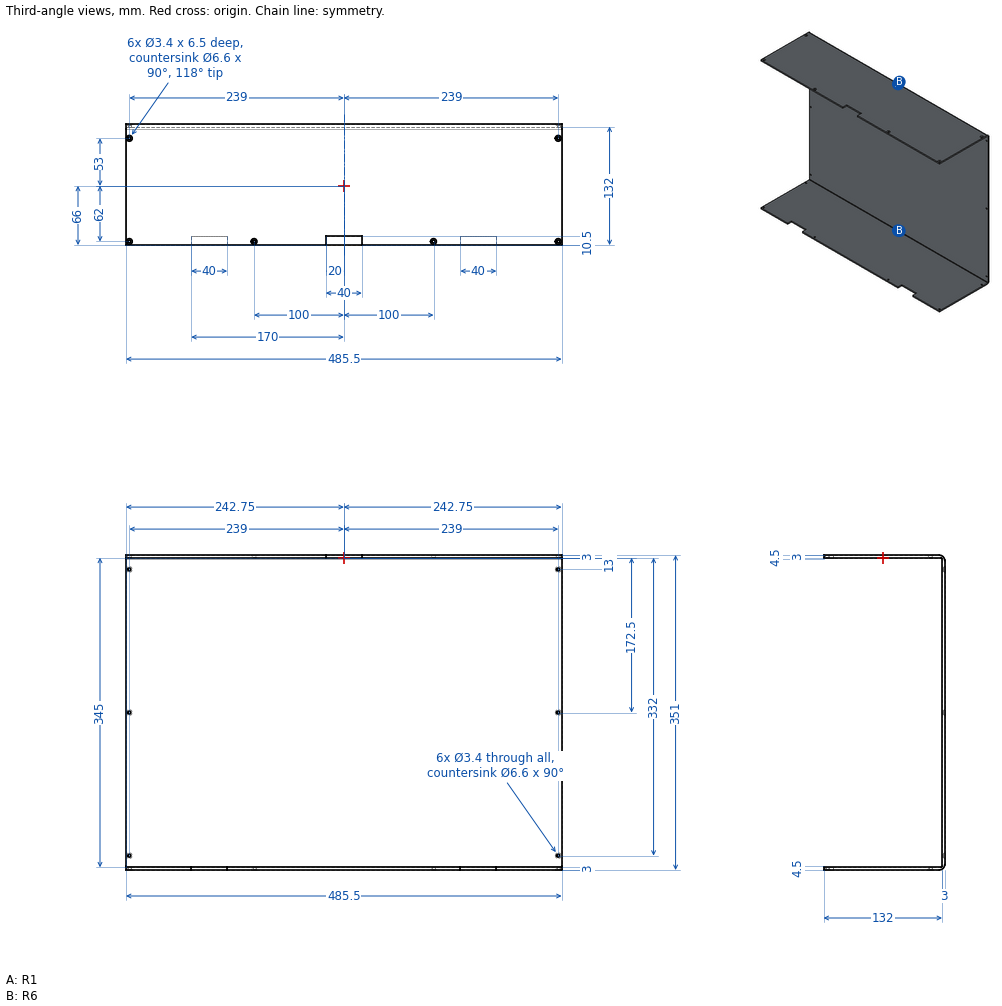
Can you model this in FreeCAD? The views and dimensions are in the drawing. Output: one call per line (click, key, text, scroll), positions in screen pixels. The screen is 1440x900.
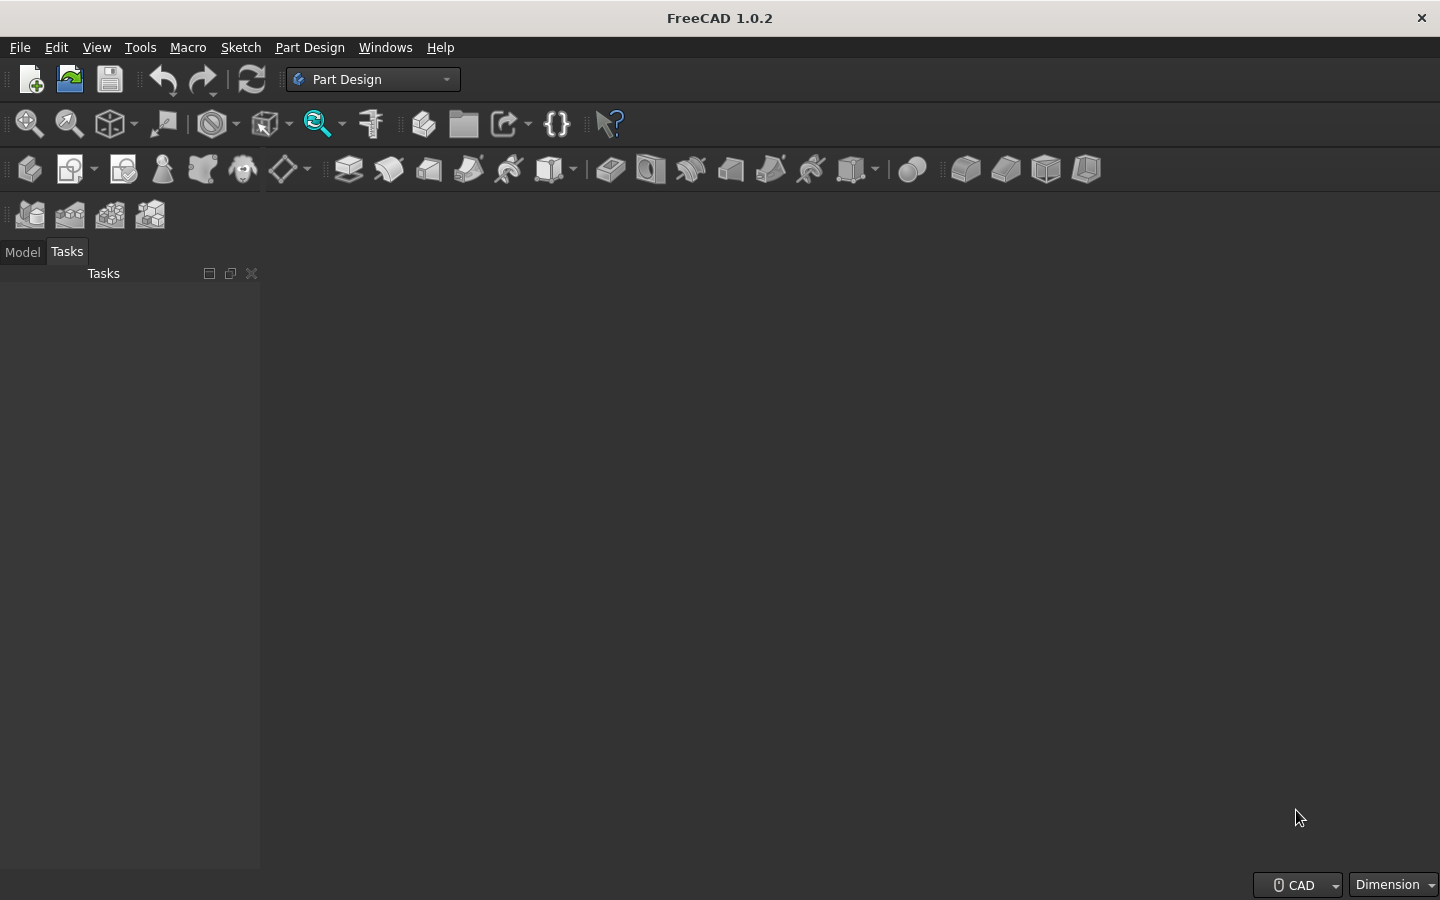
click(1214, 80)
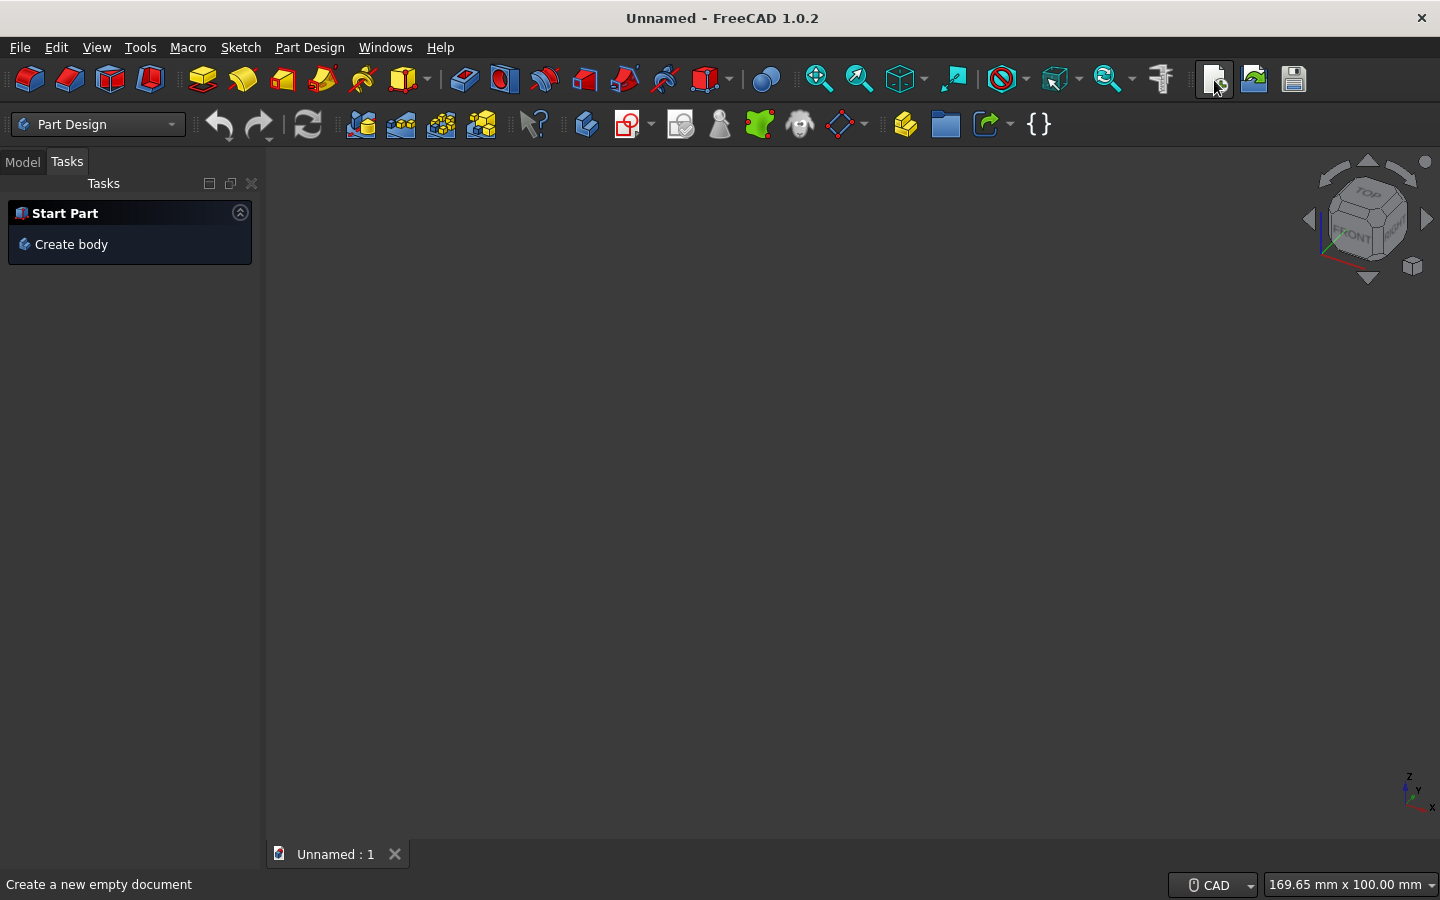
click(628, 124)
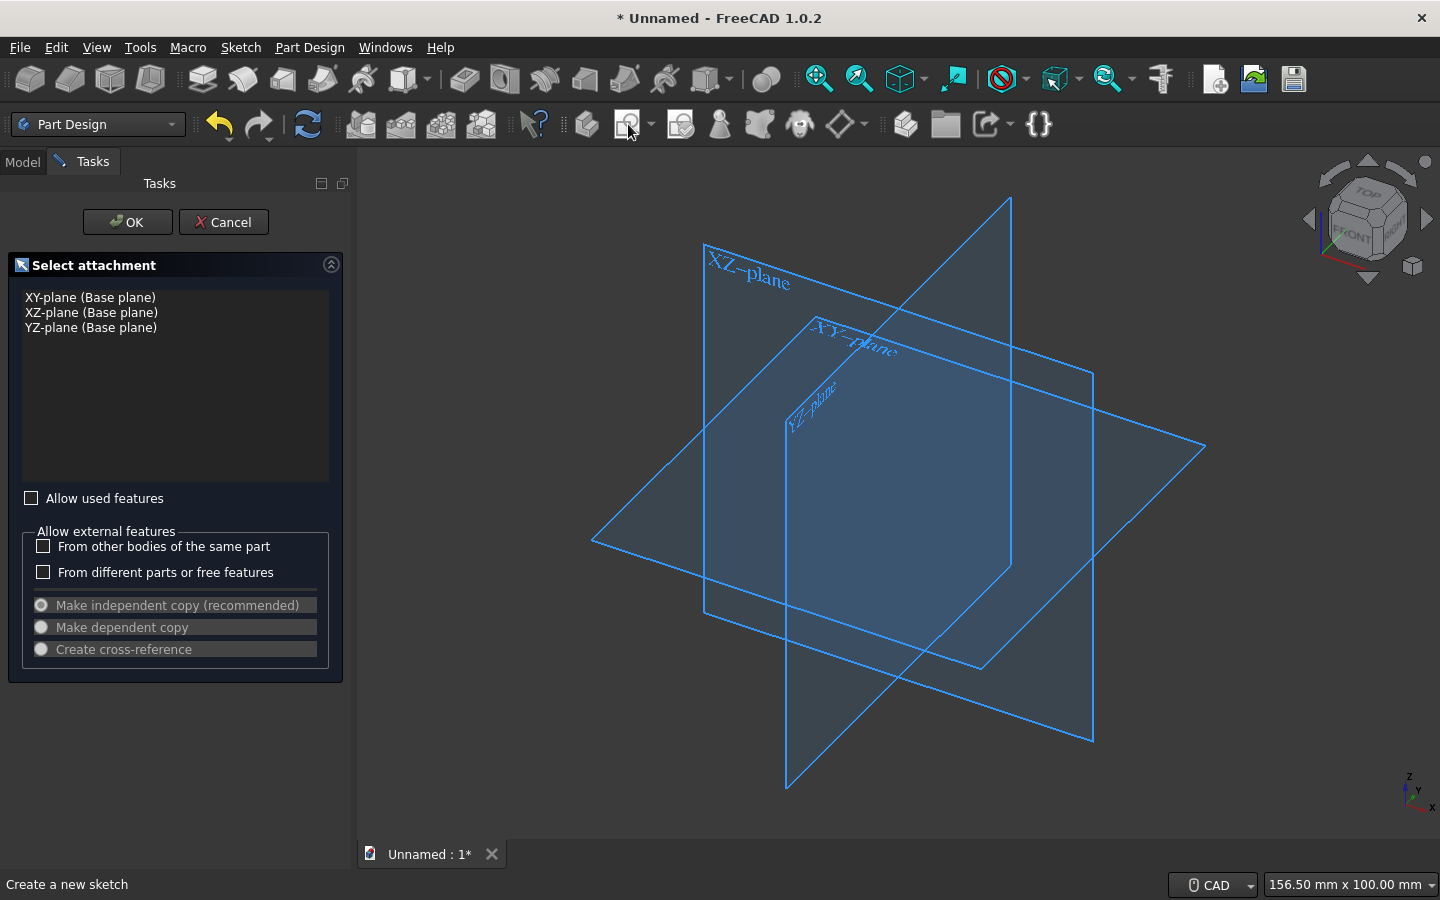
click(82, 298)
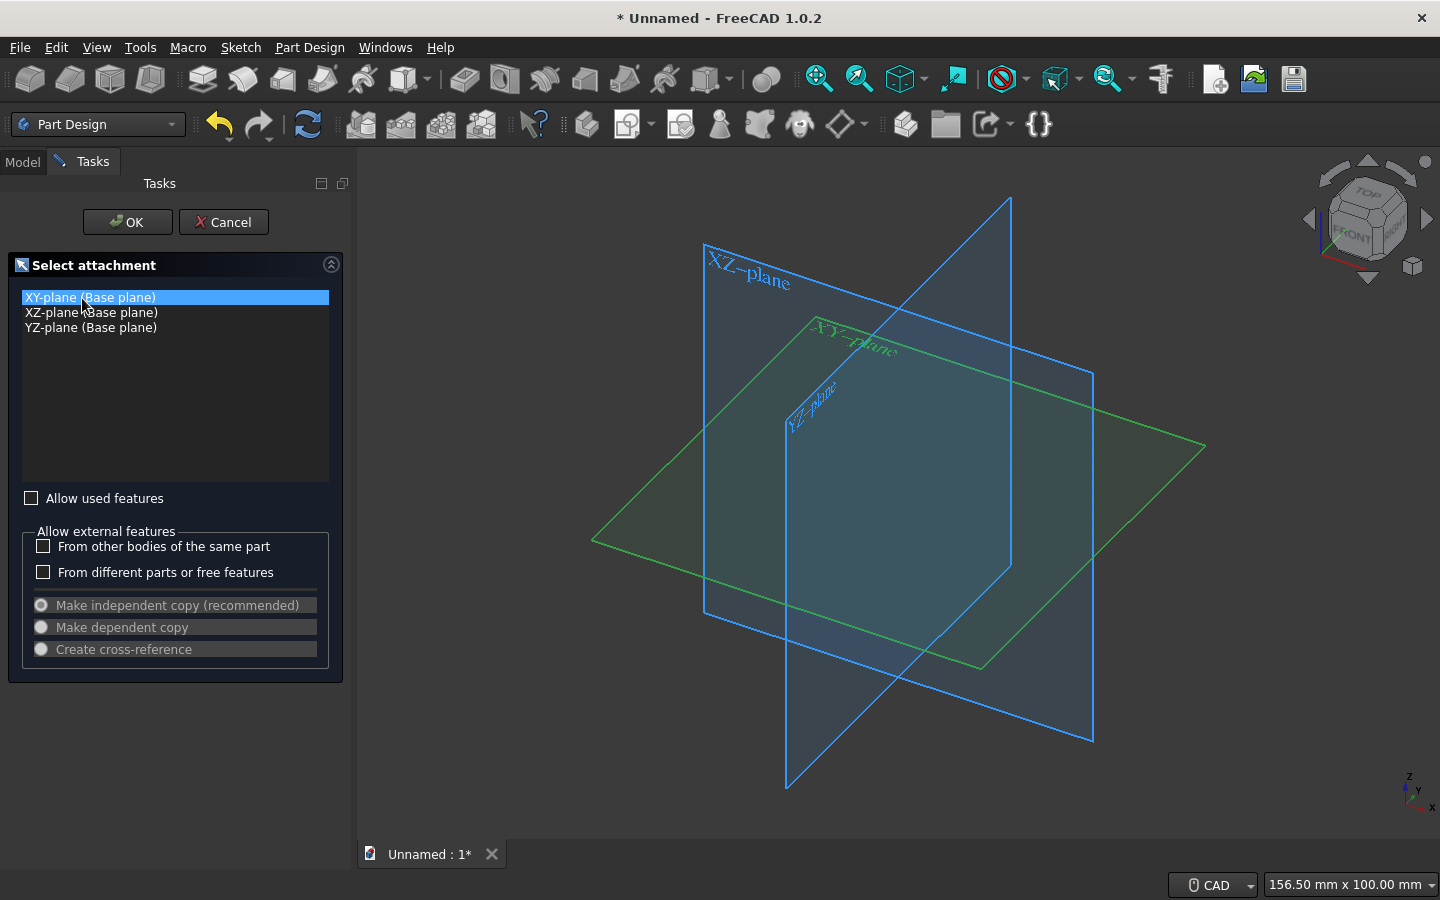
click(128, 222)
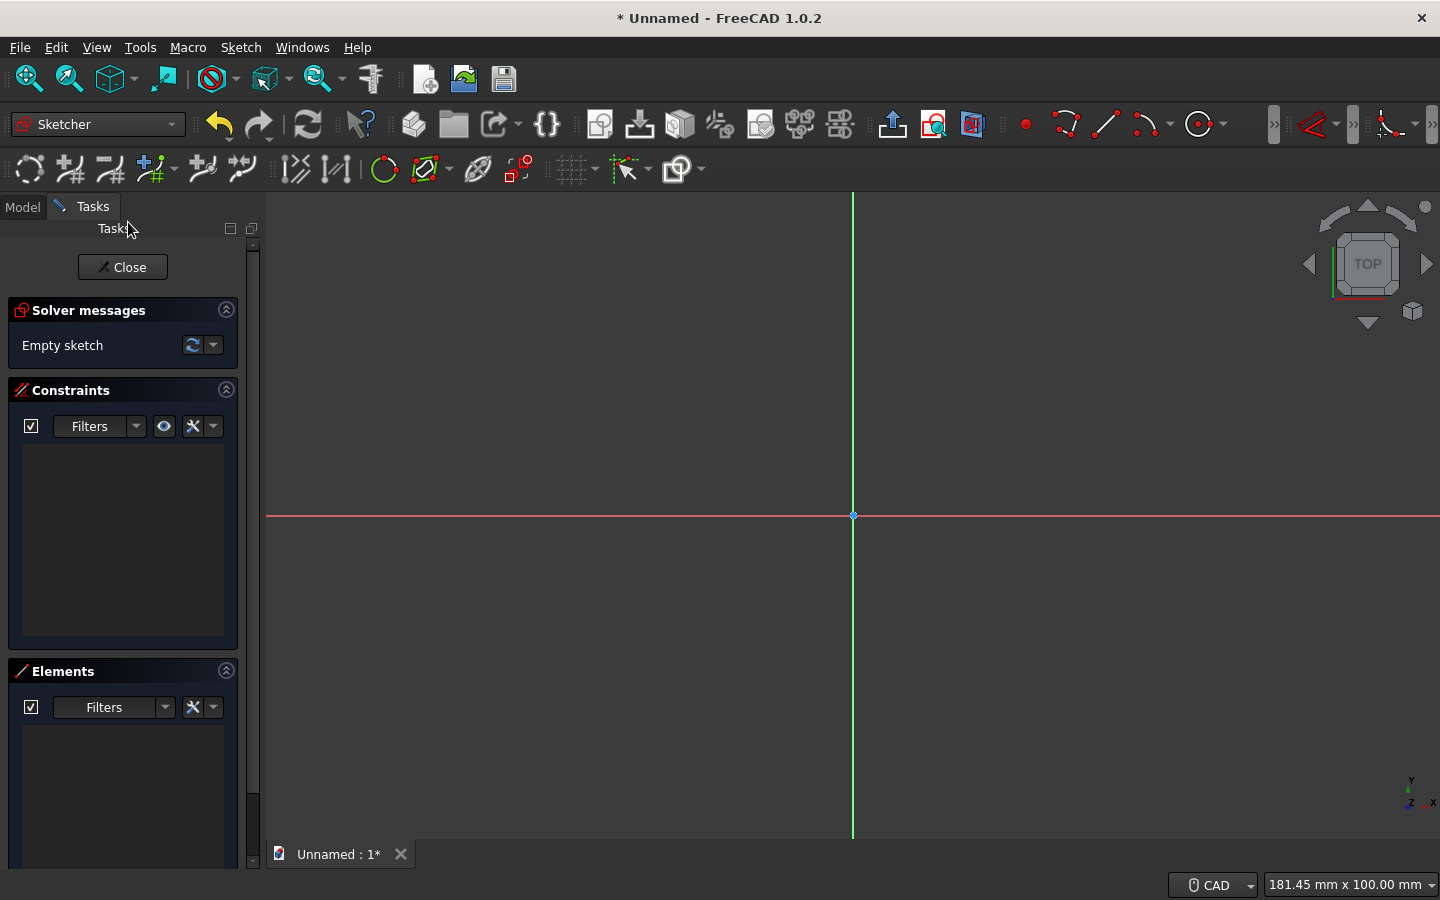
scroll(767, 515, down, 8)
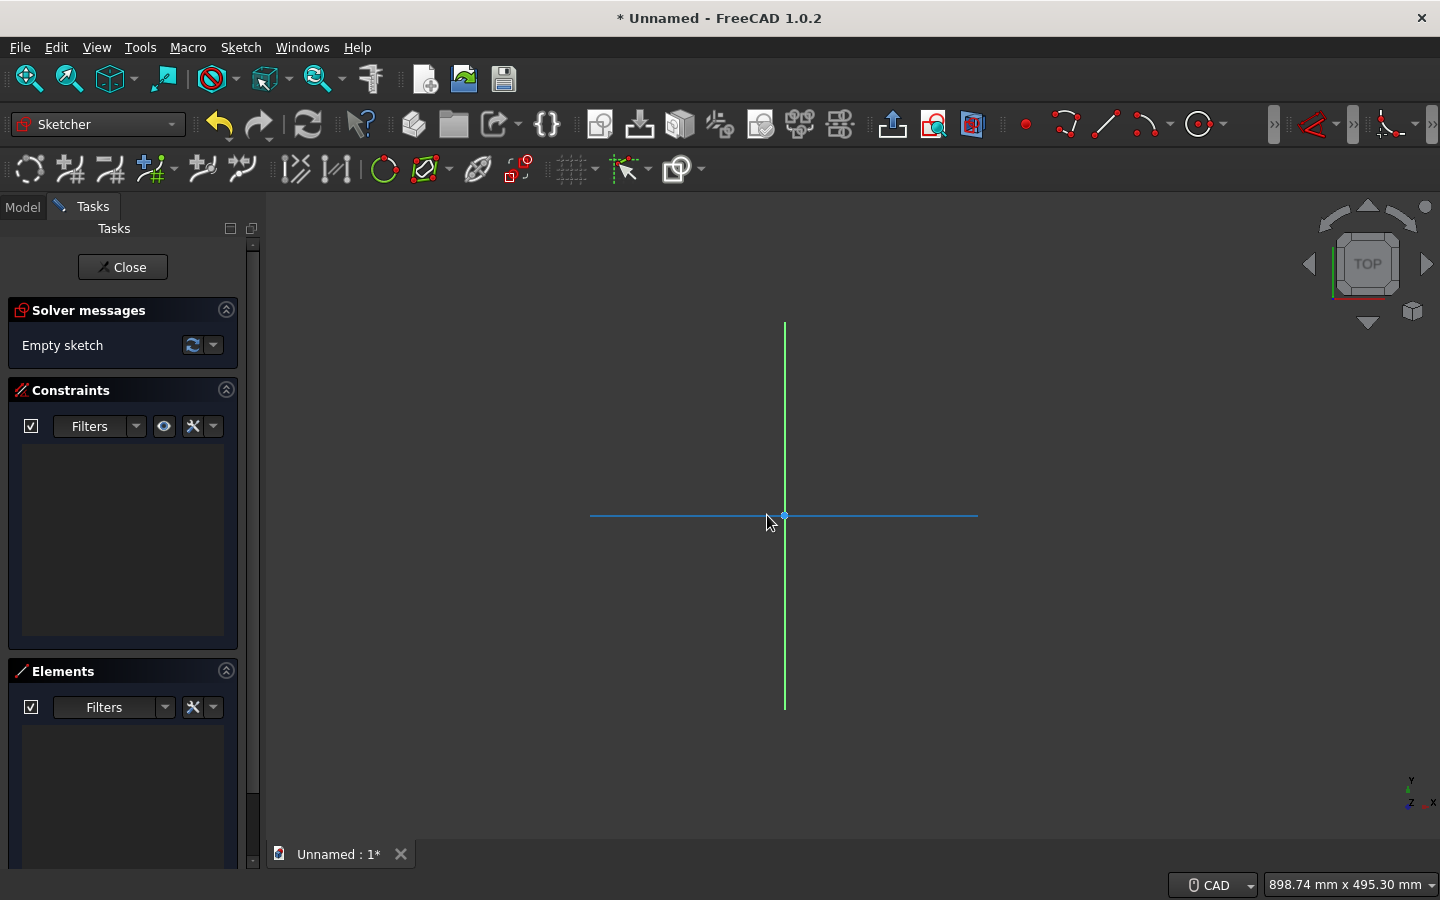
key(g)
key(v)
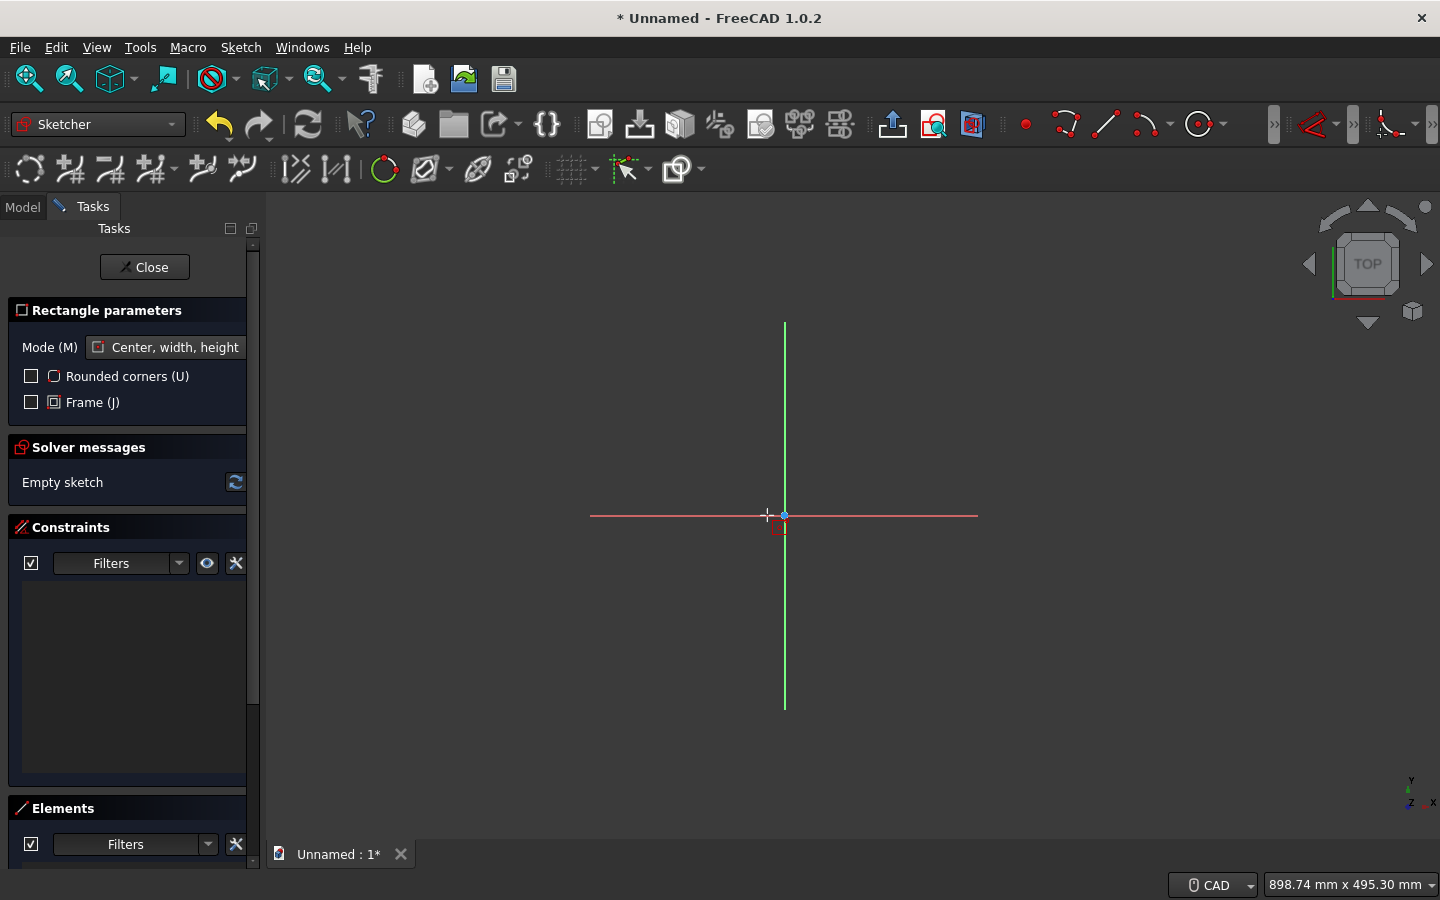
click(785, 516)
move(1102, 429)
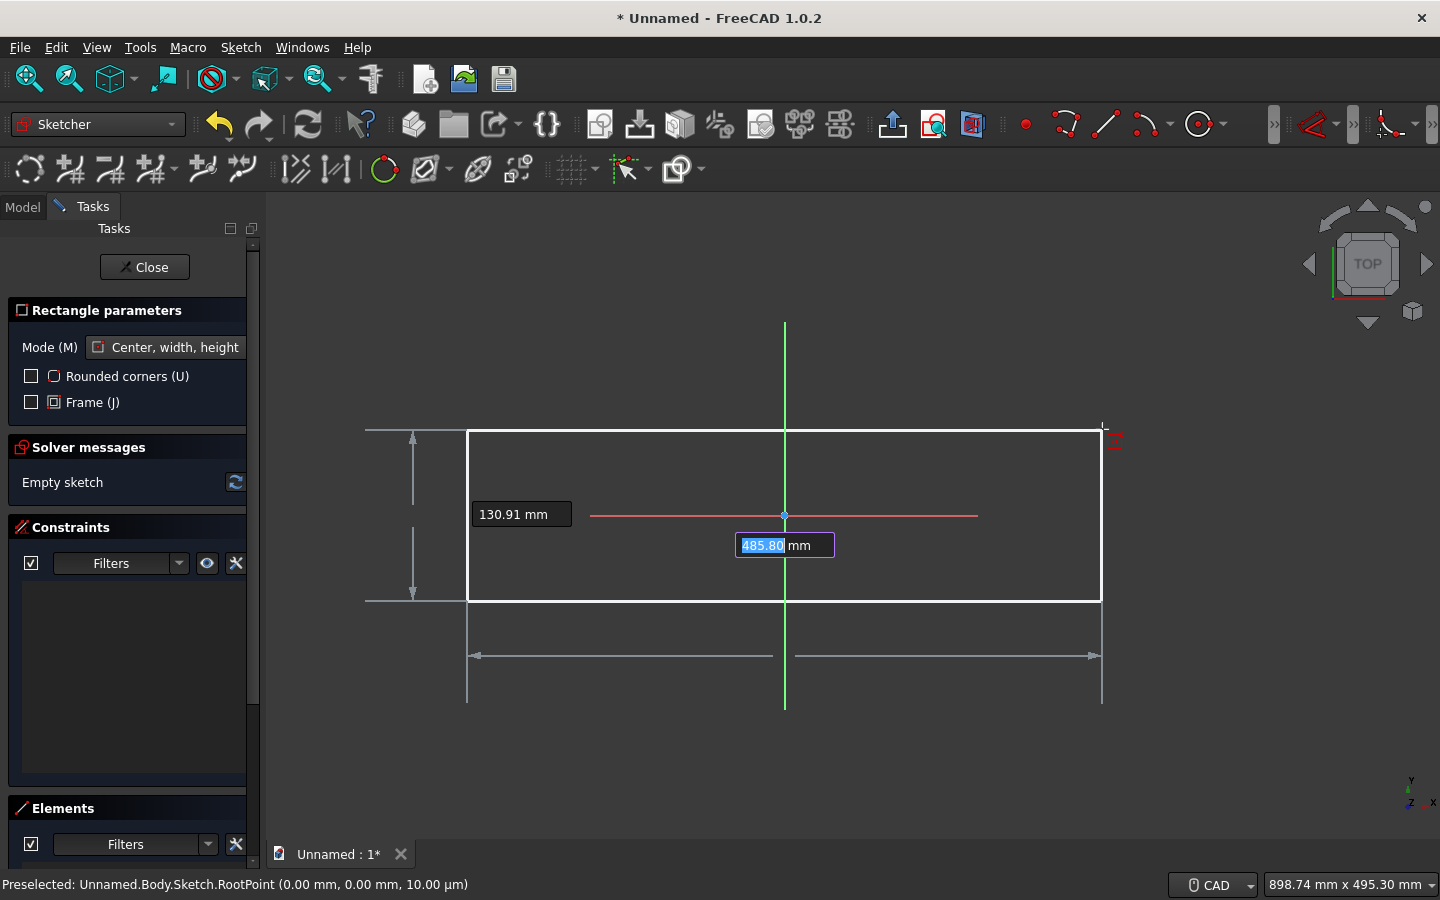
text(485.5)
key(Tab)
text(132)
key(Return)
key(Escape)